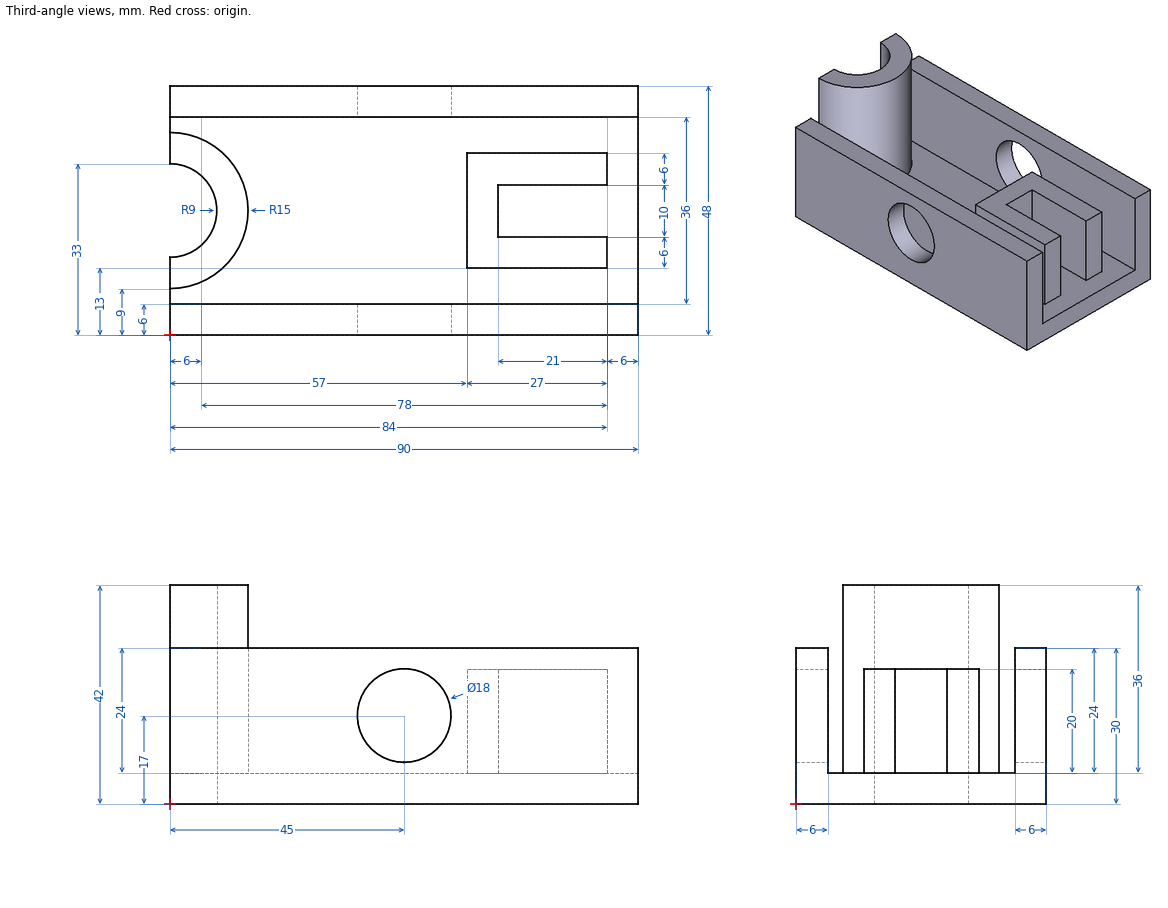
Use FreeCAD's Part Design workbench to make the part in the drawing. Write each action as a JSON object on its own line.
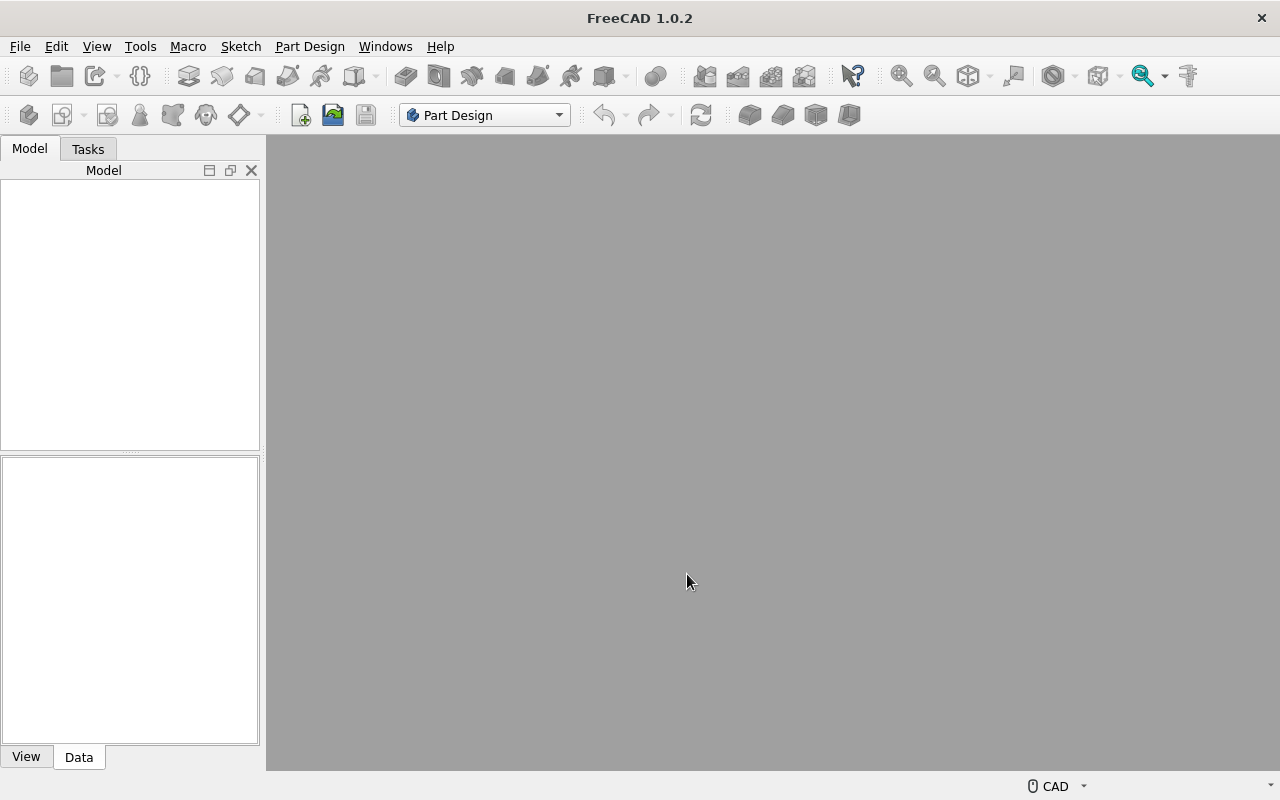
{"action": "key", "text": "ctrl+n"}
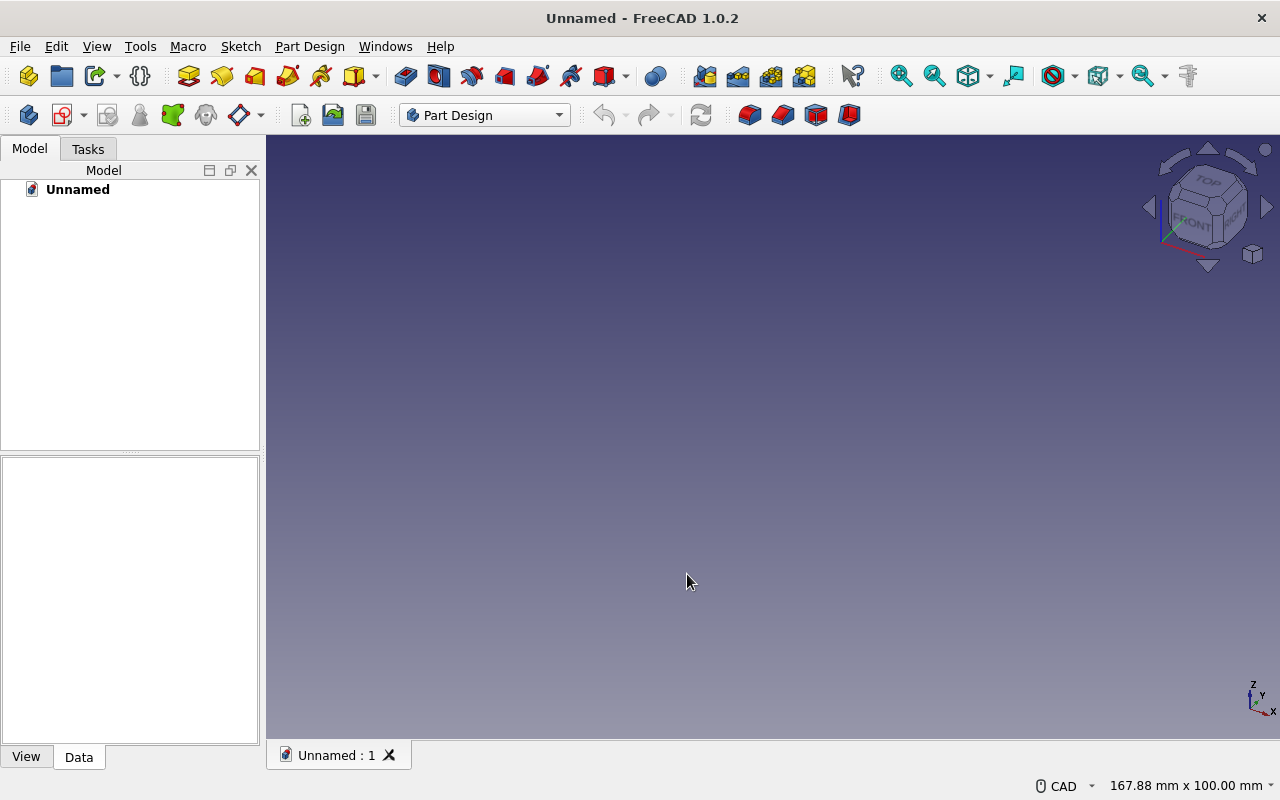
{"action": "left_click", "coordinate": [62, 116]}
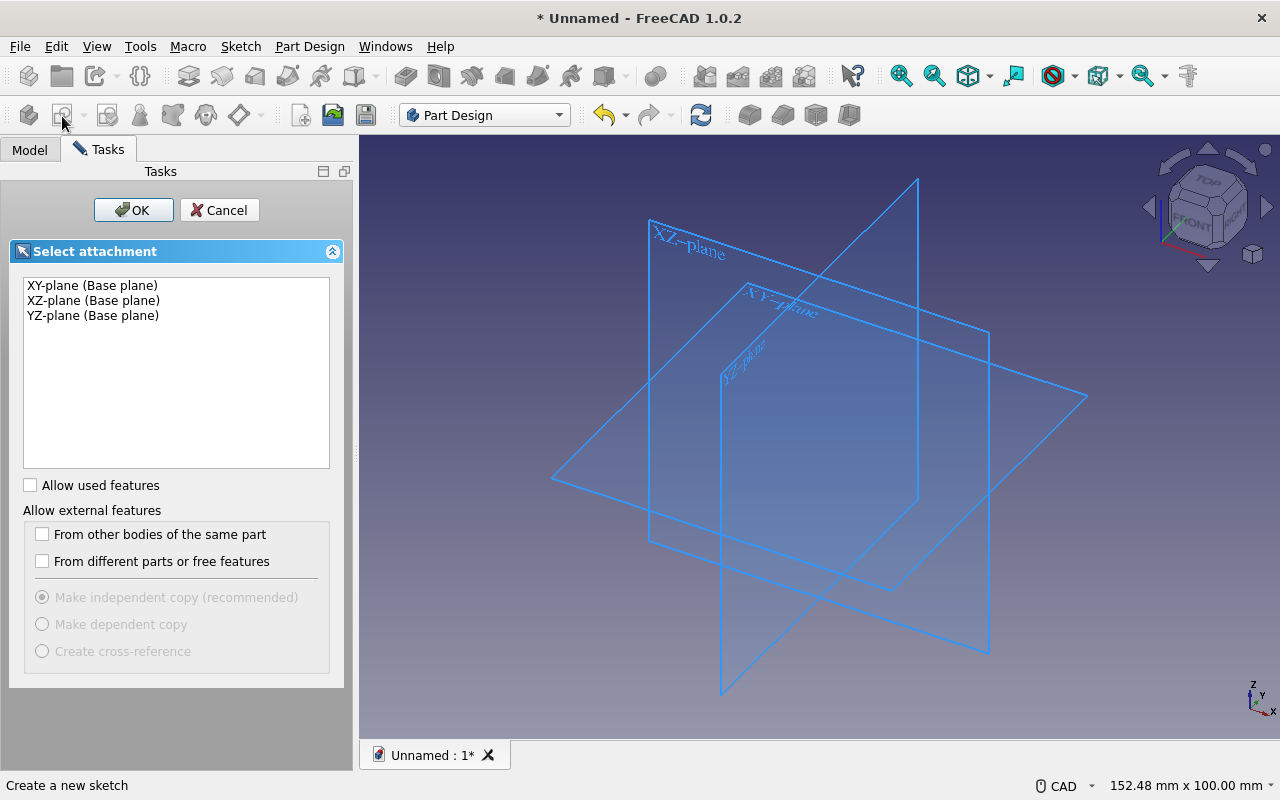
{"action": "left_click", "coordinate": [84, 286]}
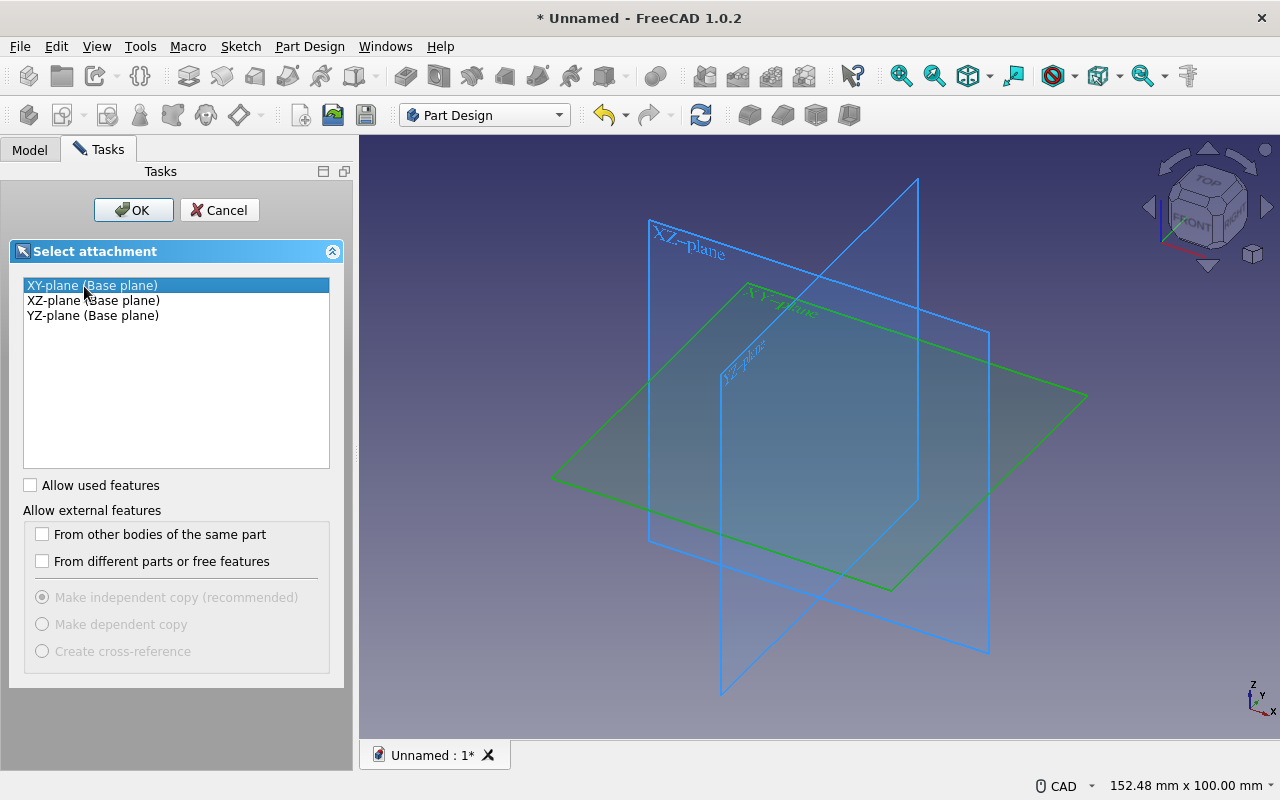
{"action": "left_click", "coordinate": [134, 210]}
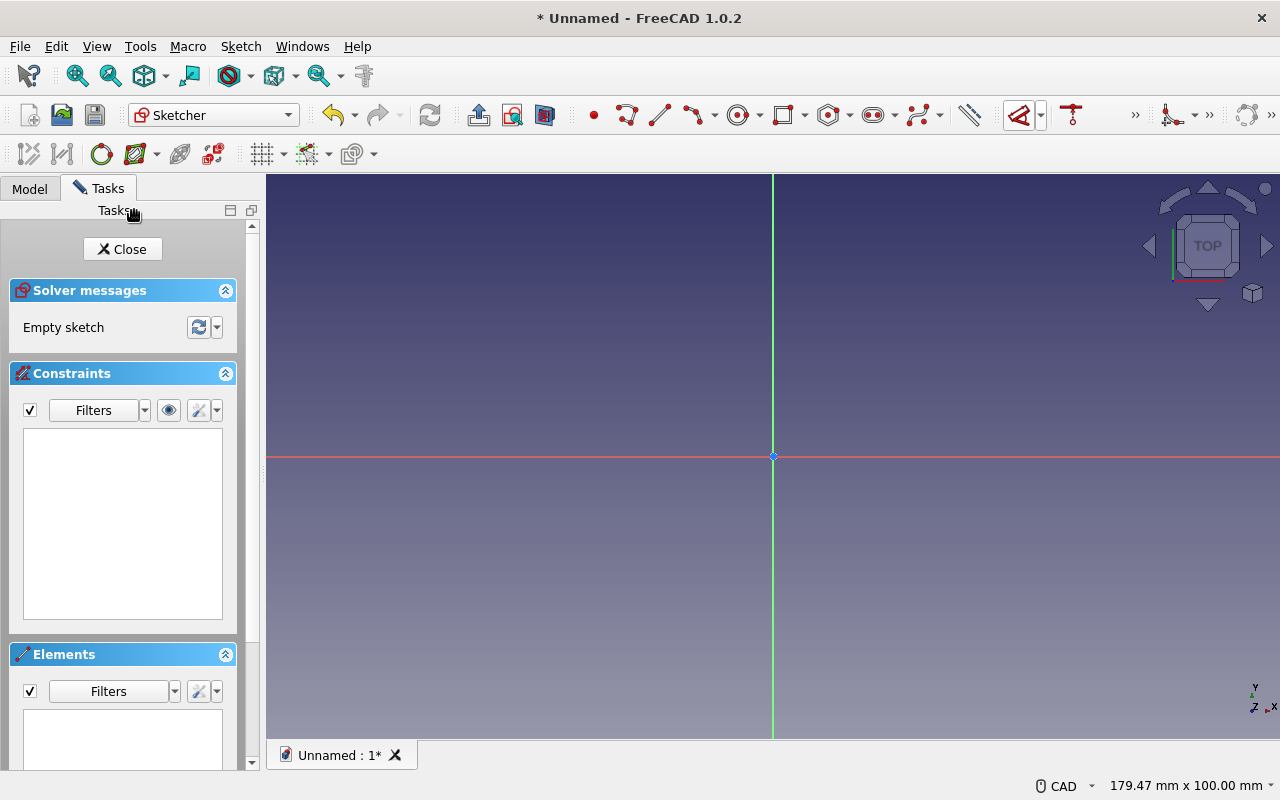
{"action": "scroll", "coordinate": [294, 711], "scroll_direction": "down", "scroll_amount": 2}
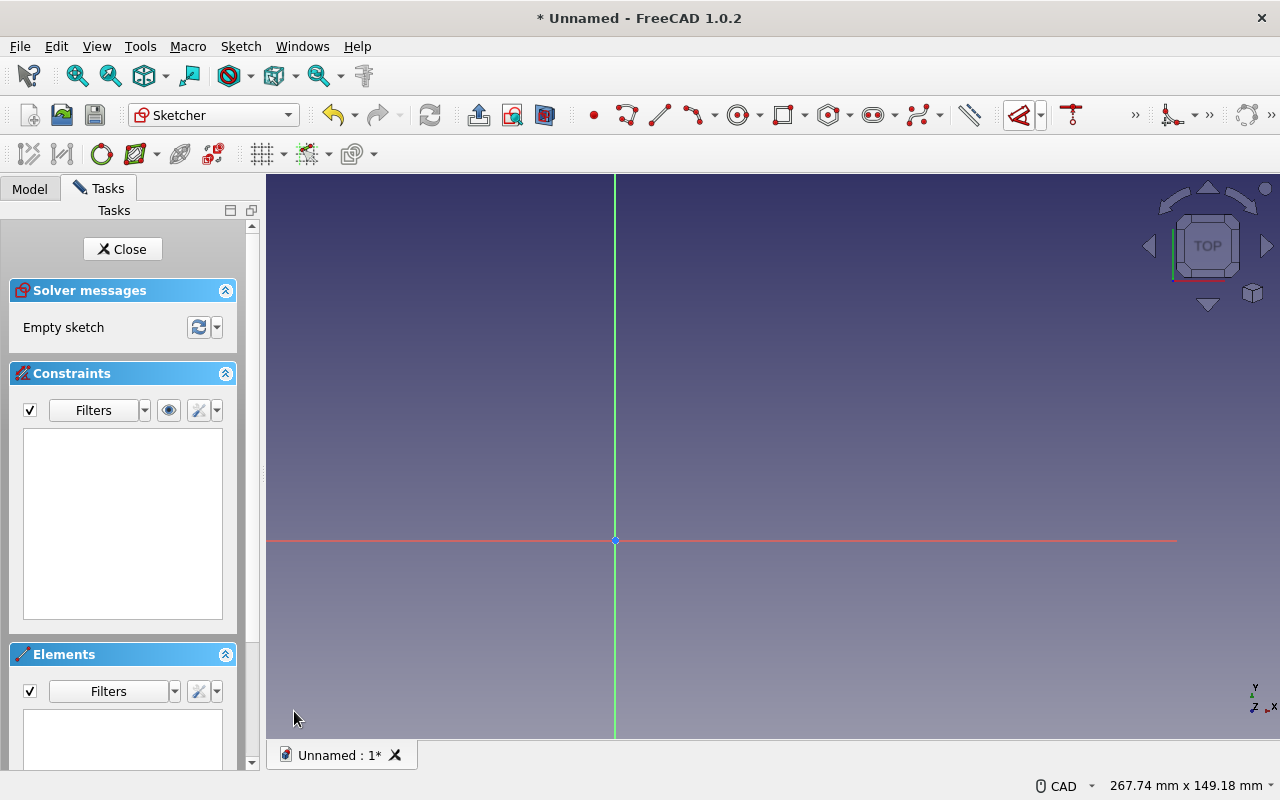
{"action": "scroll", "coordinate": [884, 442], "scroll_direction": "up", "scroll_amount": 3}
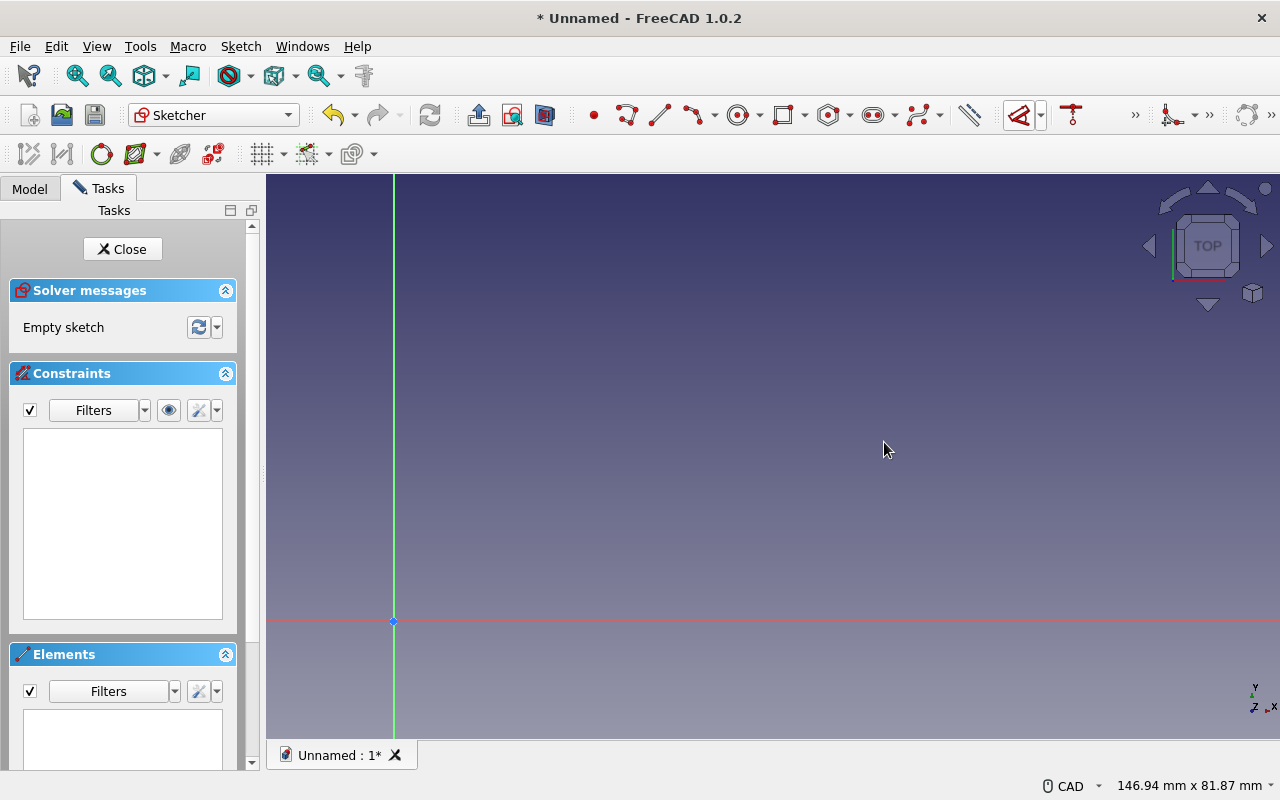
{"action": "key", "text": "g r"}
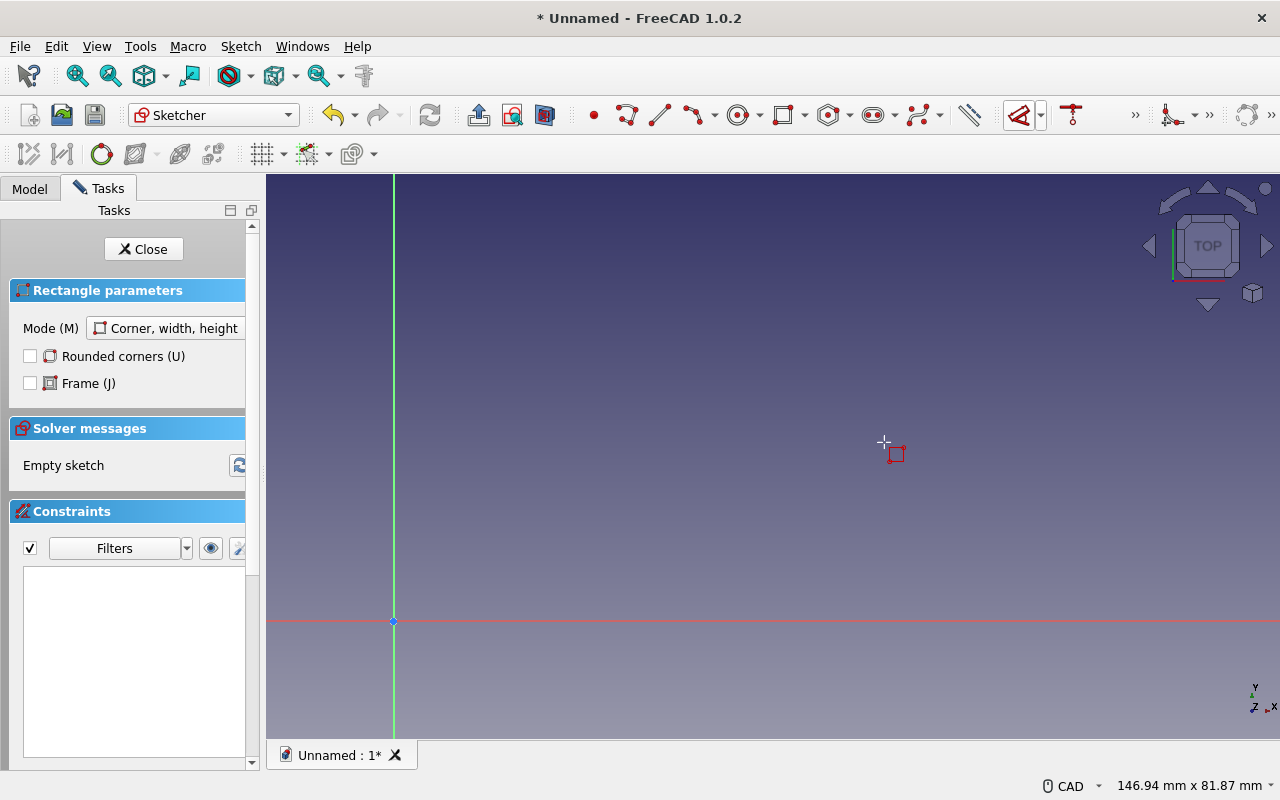
{"action": "left_click", "coordinate": [394, 621]}
{"action": "mouse_move", "coordinate": [1015, 290]}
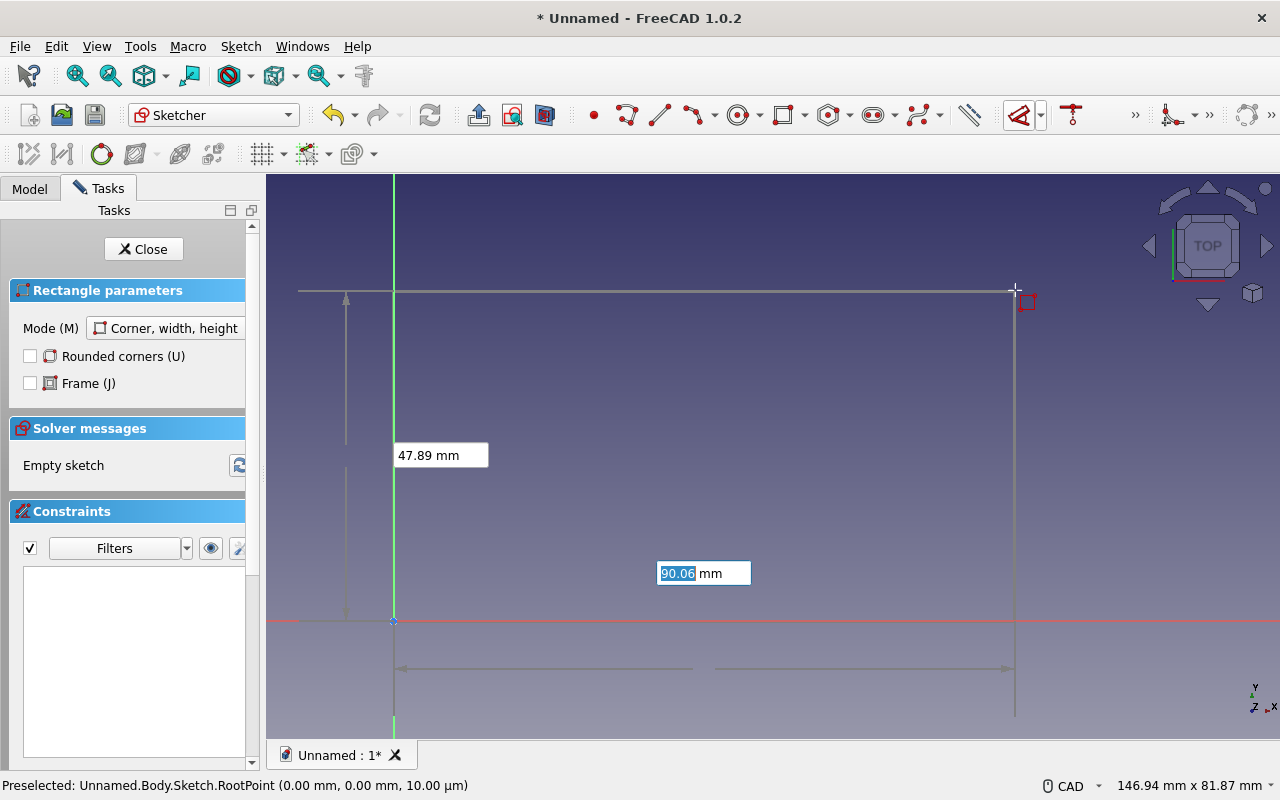
{"action": "type", "text": "90"}
{"action": "key", "text": "Tab"}
{"action": "type", "text": "48"}
{"action": "key", "text": "Return"}
{"action": "key", "text": "Escape"}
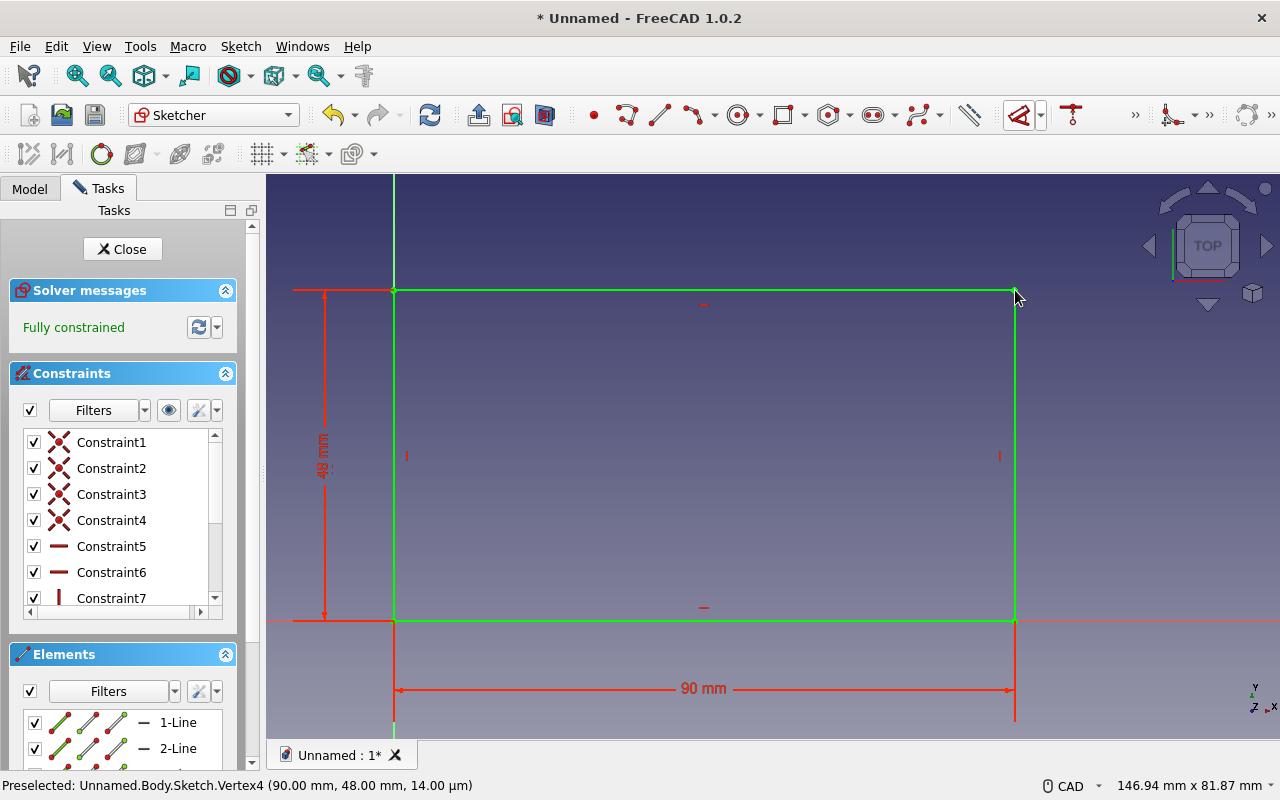
{"action": "left_click", "coordinate": [123, 249]}